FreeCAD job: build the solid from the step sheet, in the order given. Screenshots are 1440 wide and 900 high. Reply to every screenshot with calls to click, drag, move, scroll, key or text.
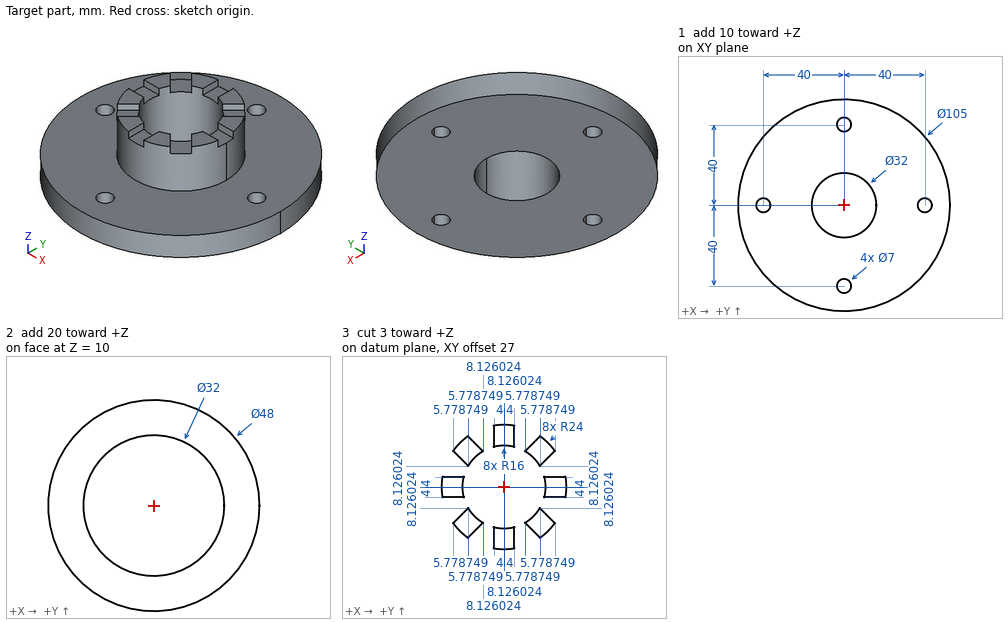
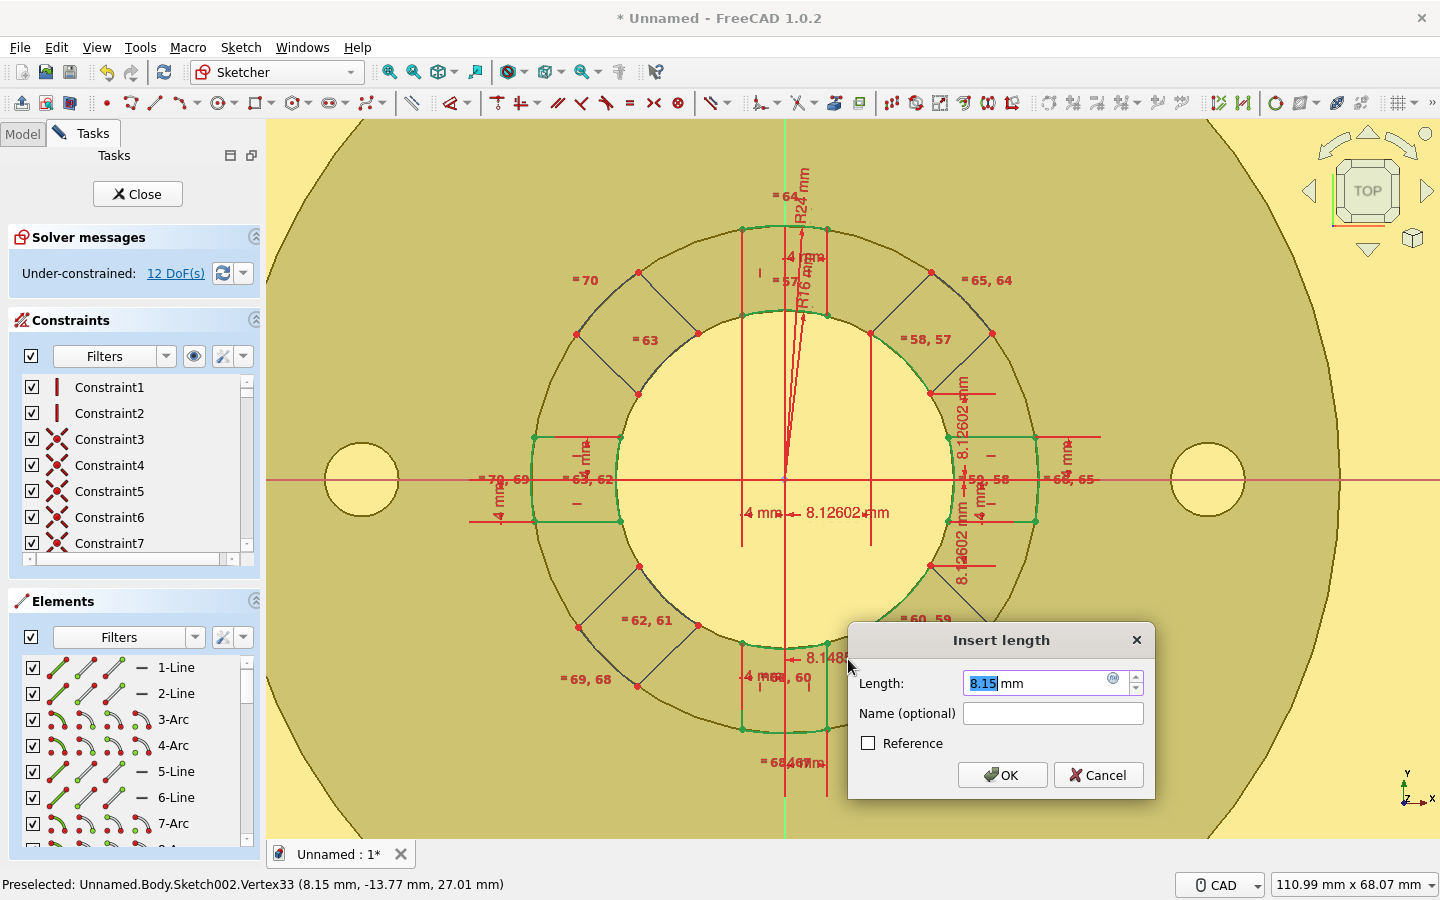
text(8.126024)
key(Return)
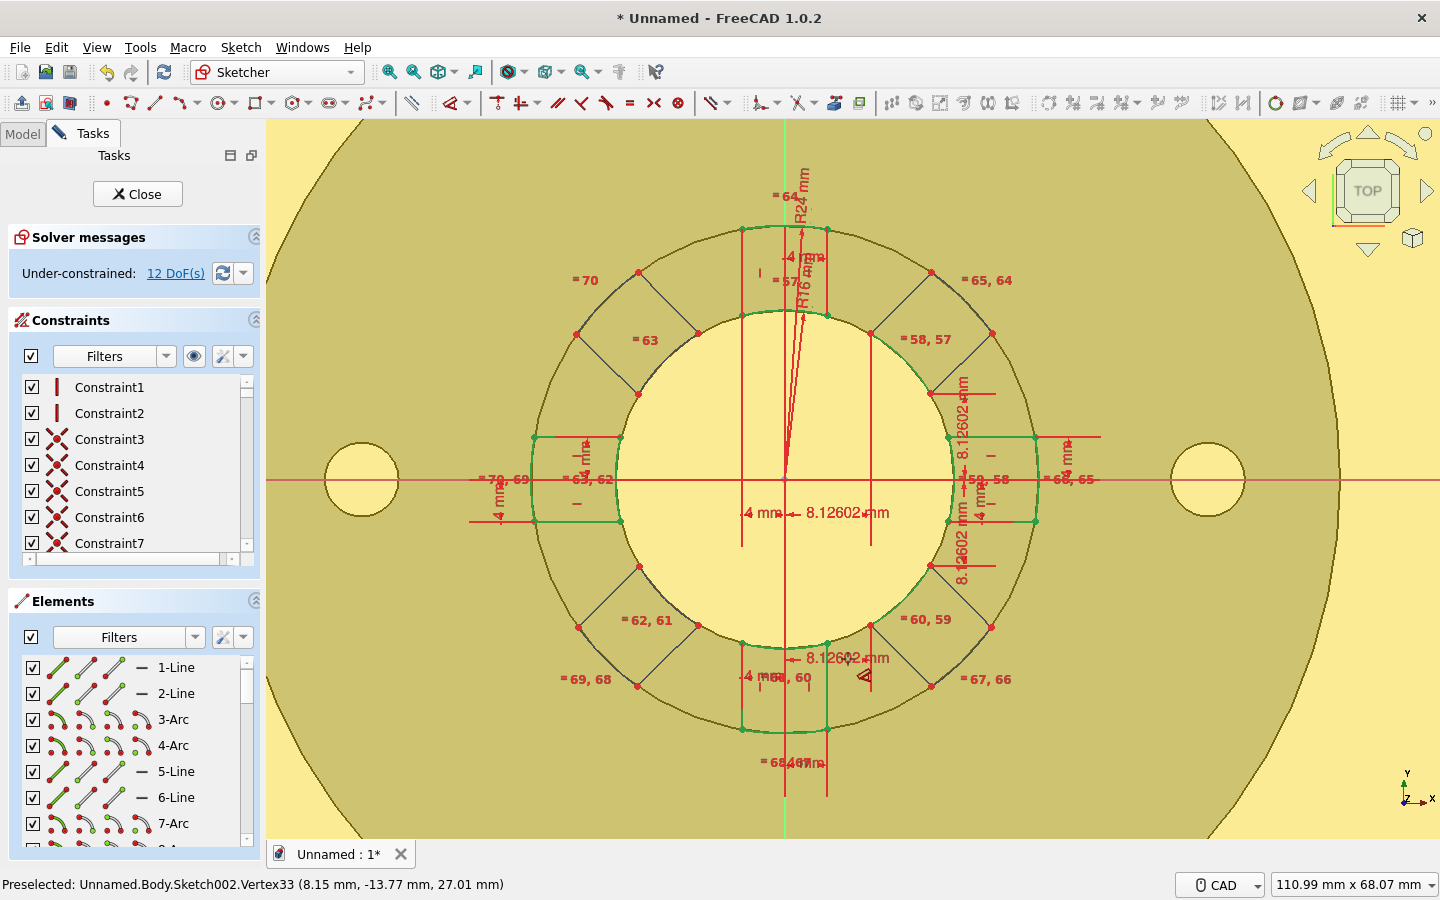
click(699, 625)
click(742, 446)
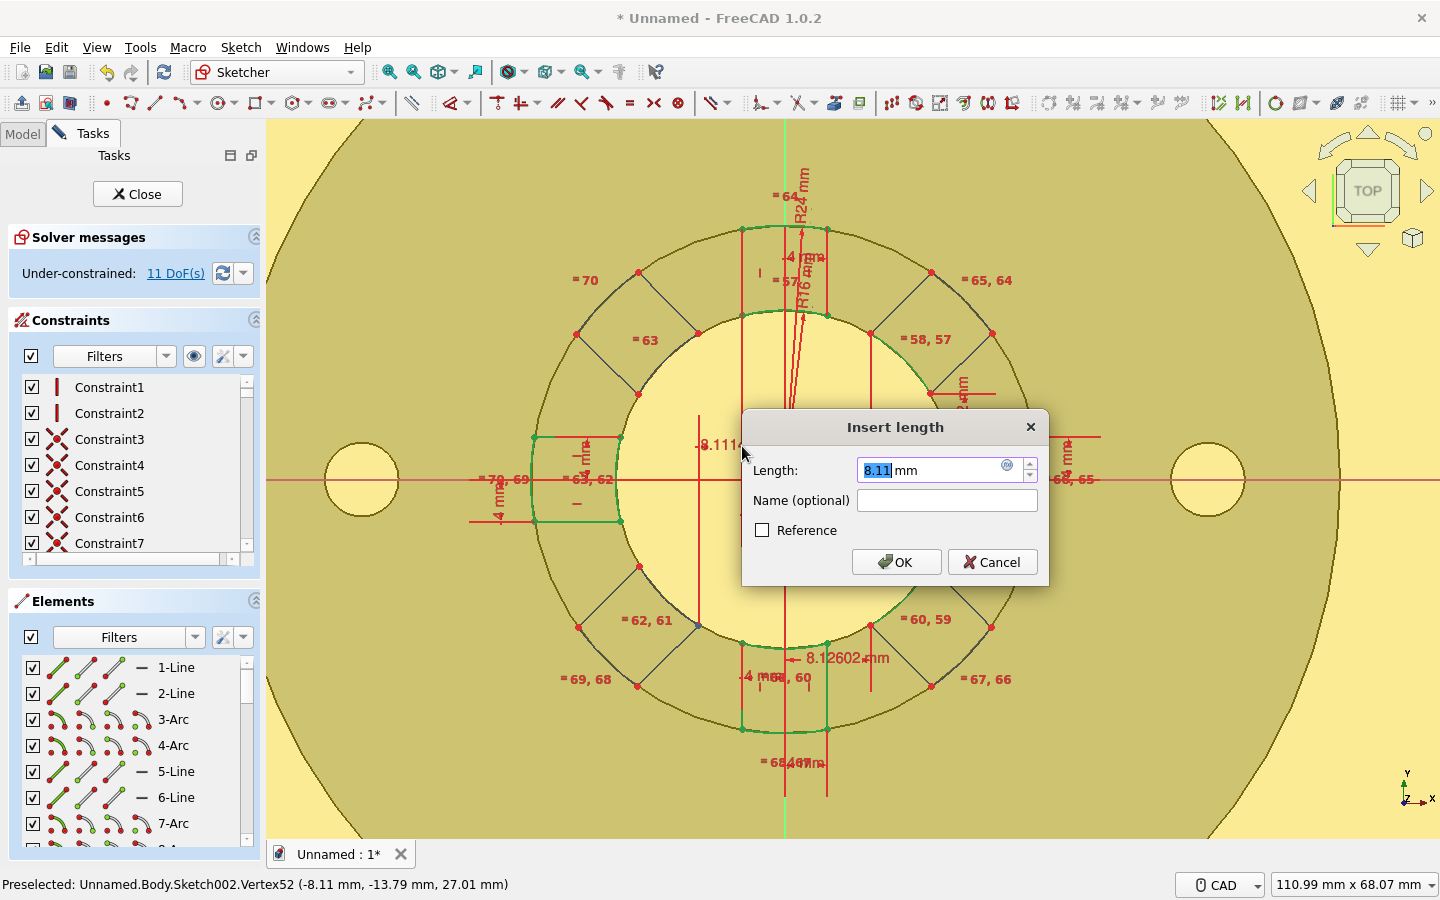
text(8.126024)
key(Return)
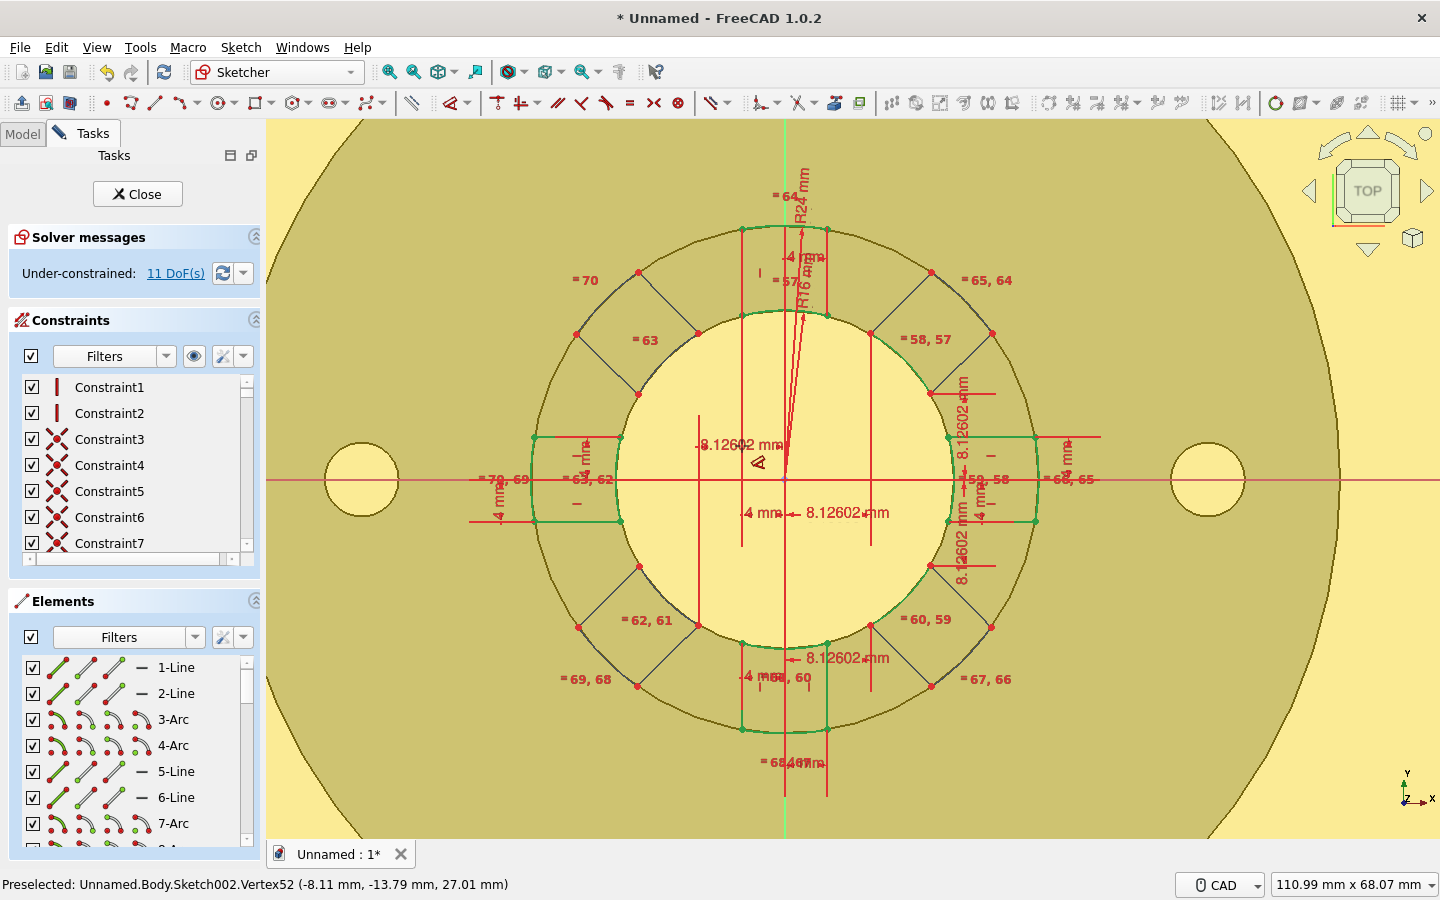
click(640, 566)
click(606, 543)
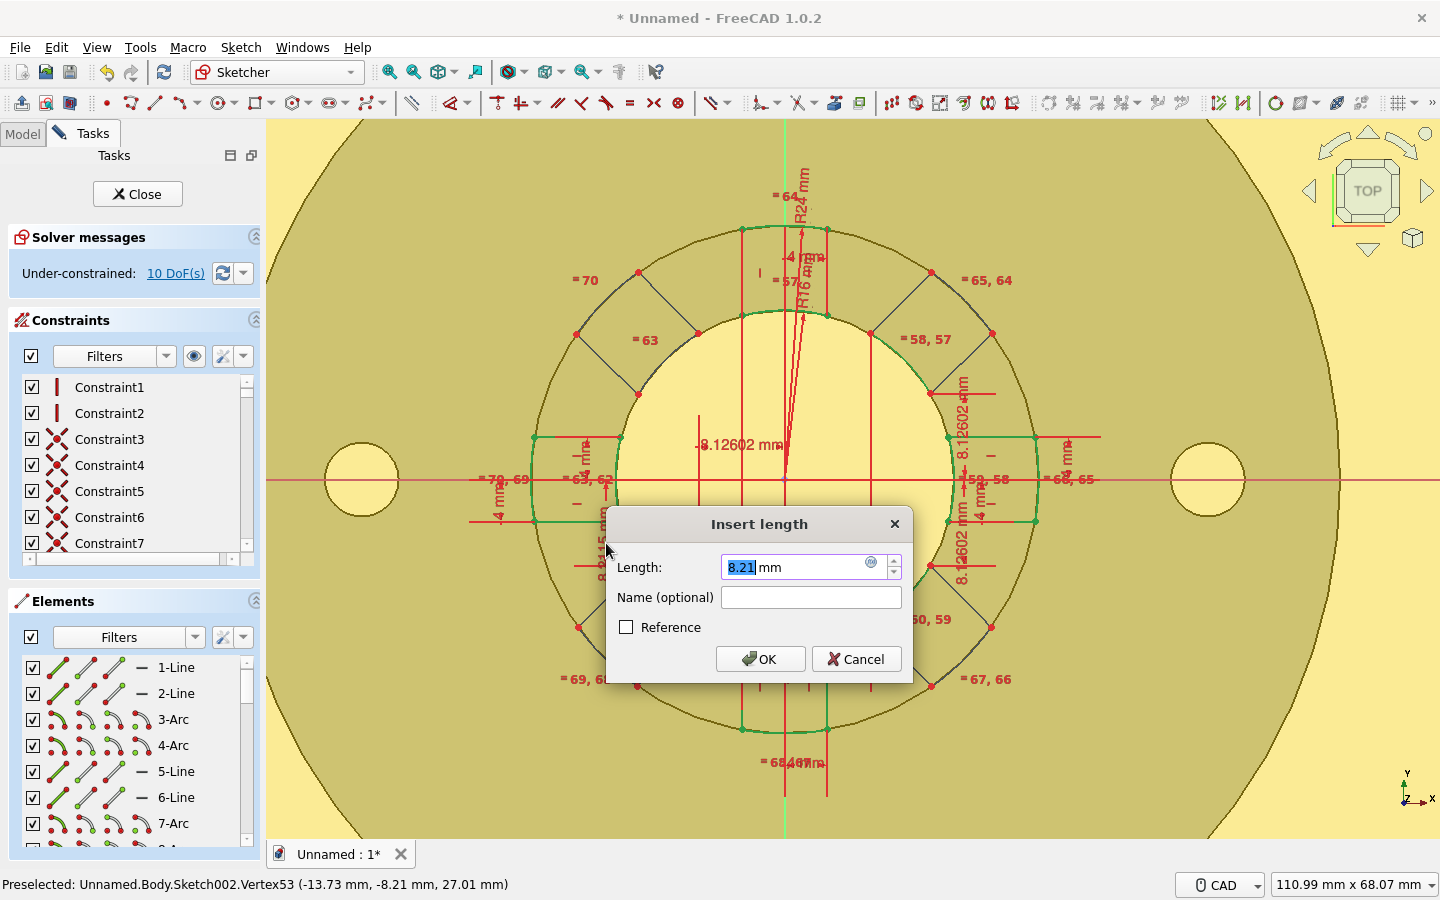
text(8.126024)
key(Return)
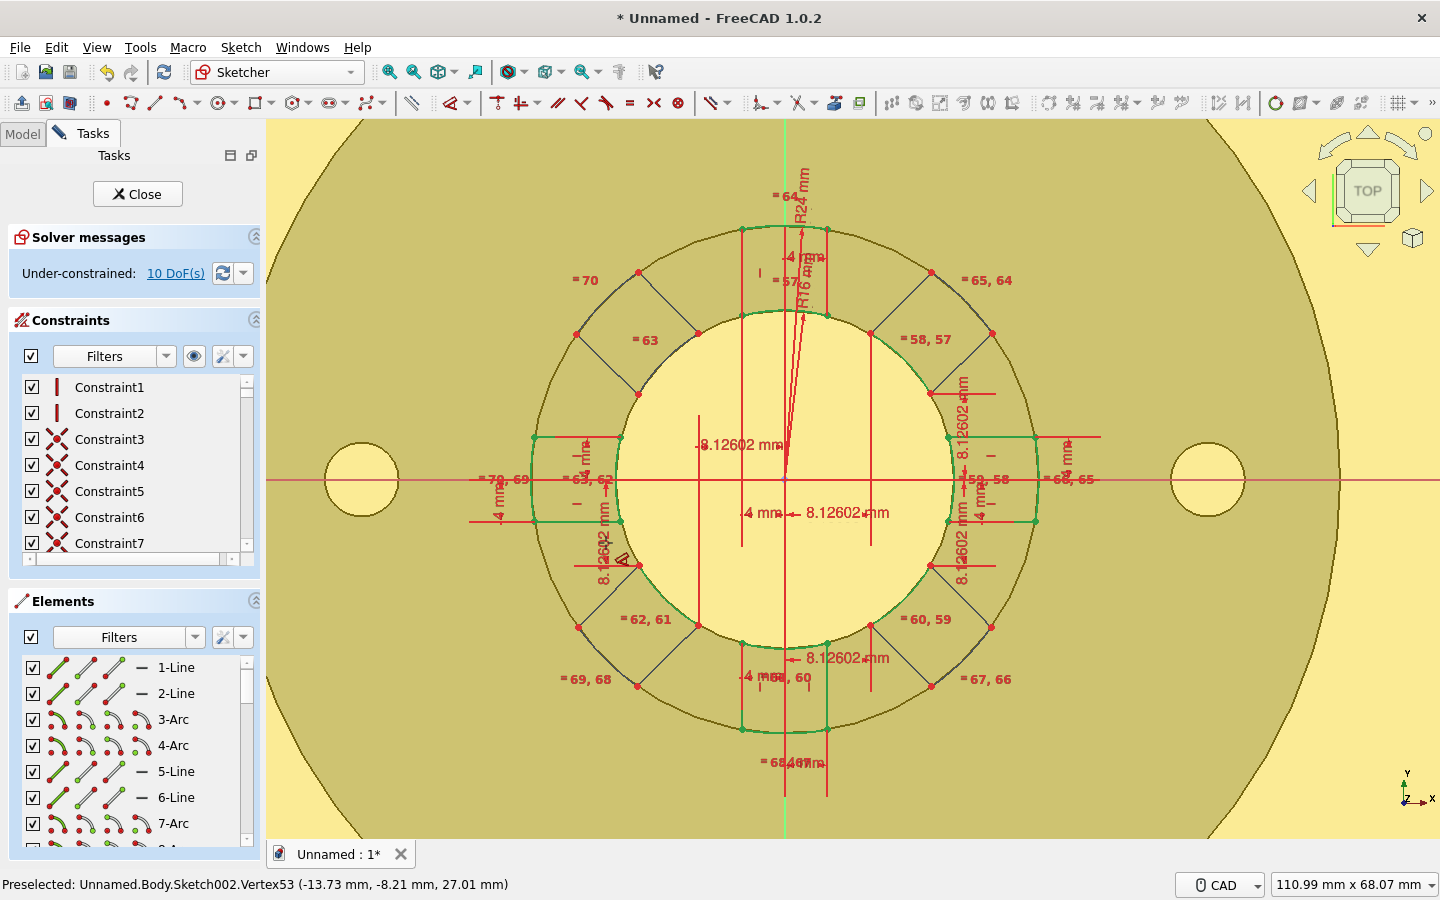
click(638, 395)
click(604, 418)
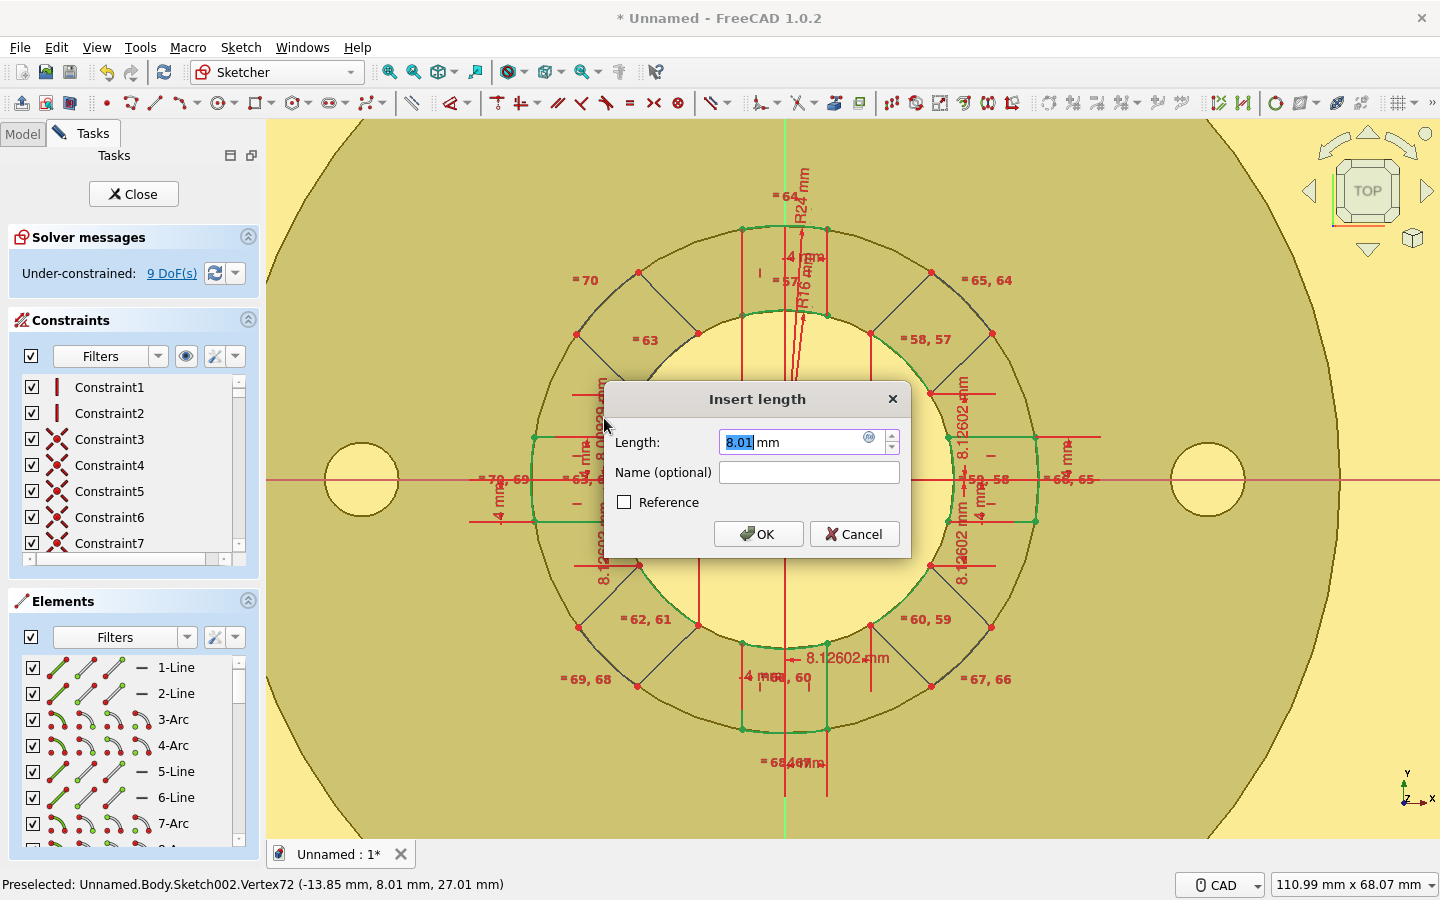
text(8.126024)
key(Return)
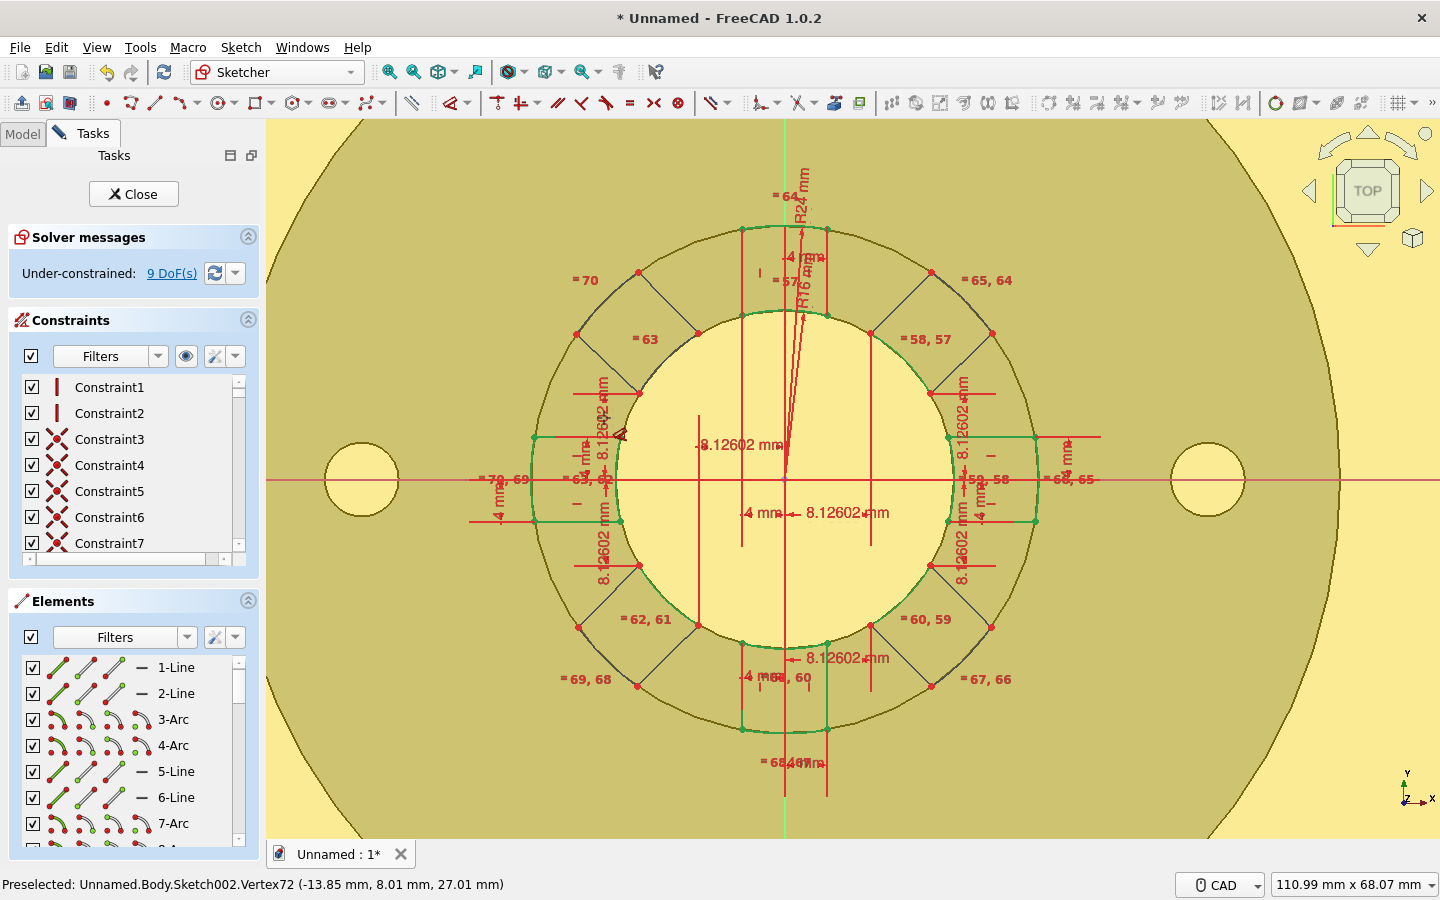
click(699, 334)
click(722, 300)